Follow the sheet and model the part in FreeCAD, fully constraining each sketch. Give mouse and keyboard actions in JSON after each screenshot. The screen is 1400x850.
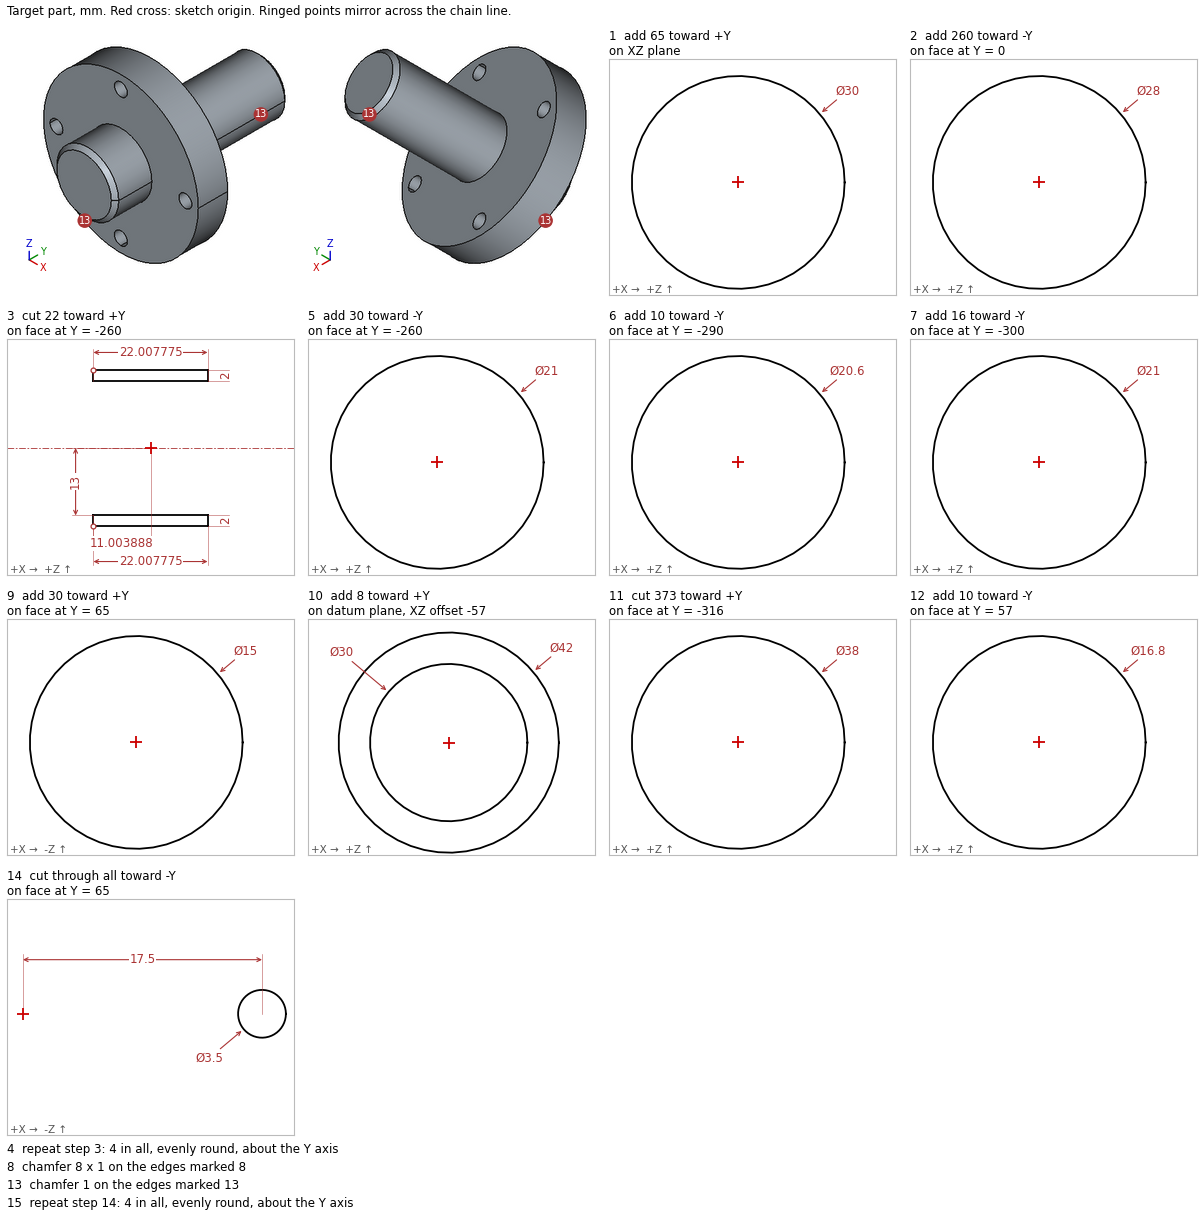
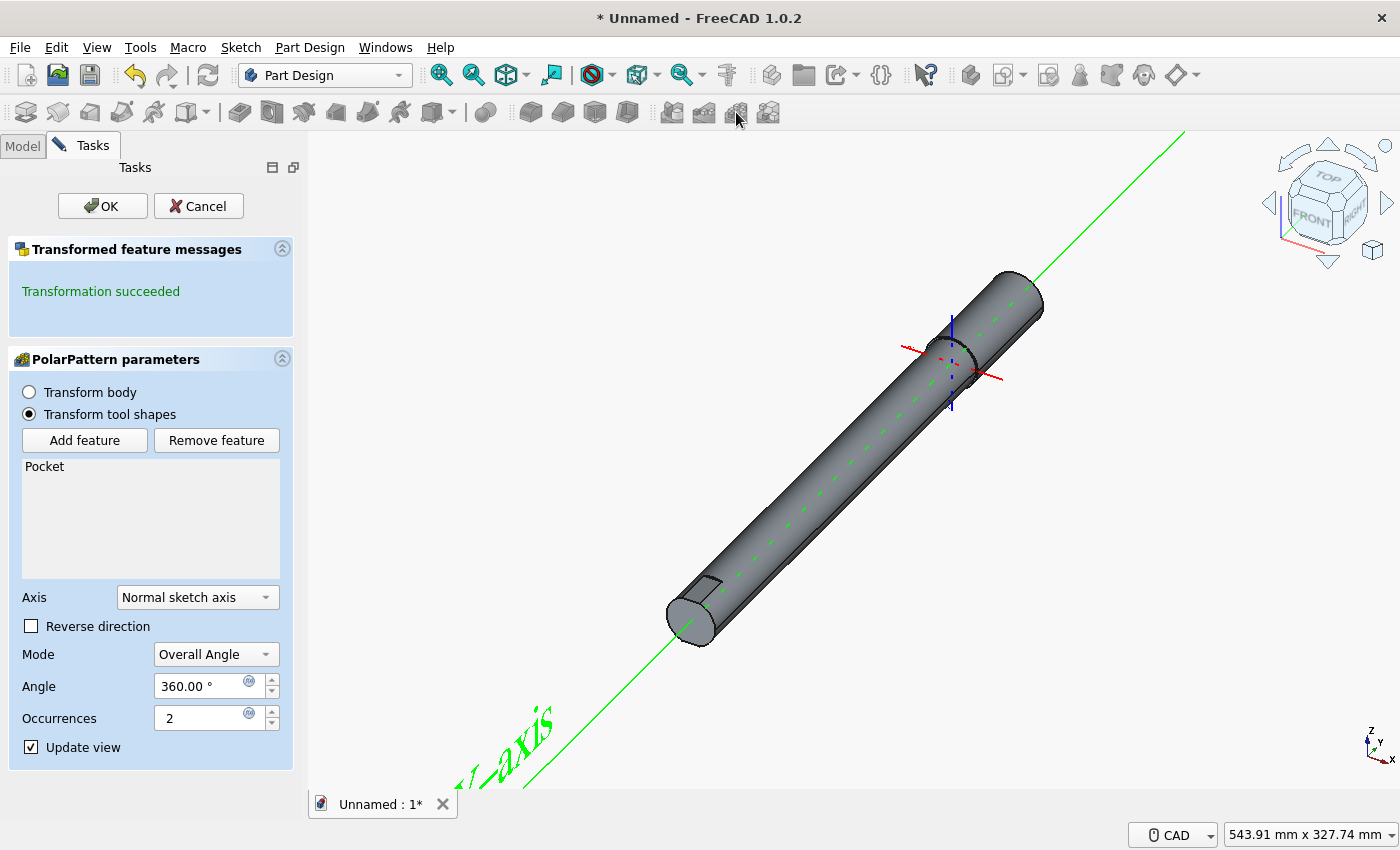
{"action": "left_click", "coordinate": [198, 598]}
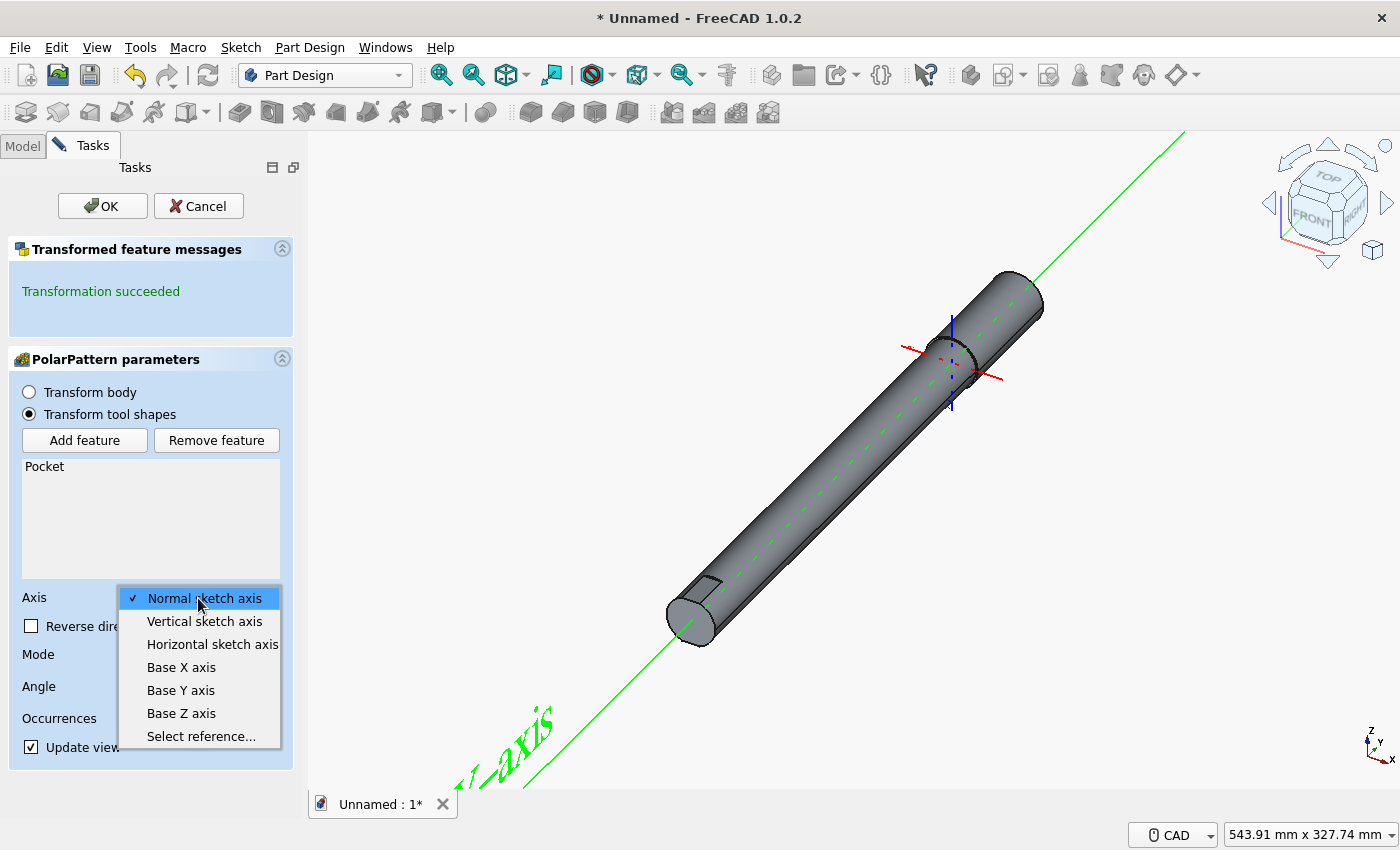
{"action": "left_click", "coordinate": [198, 690]}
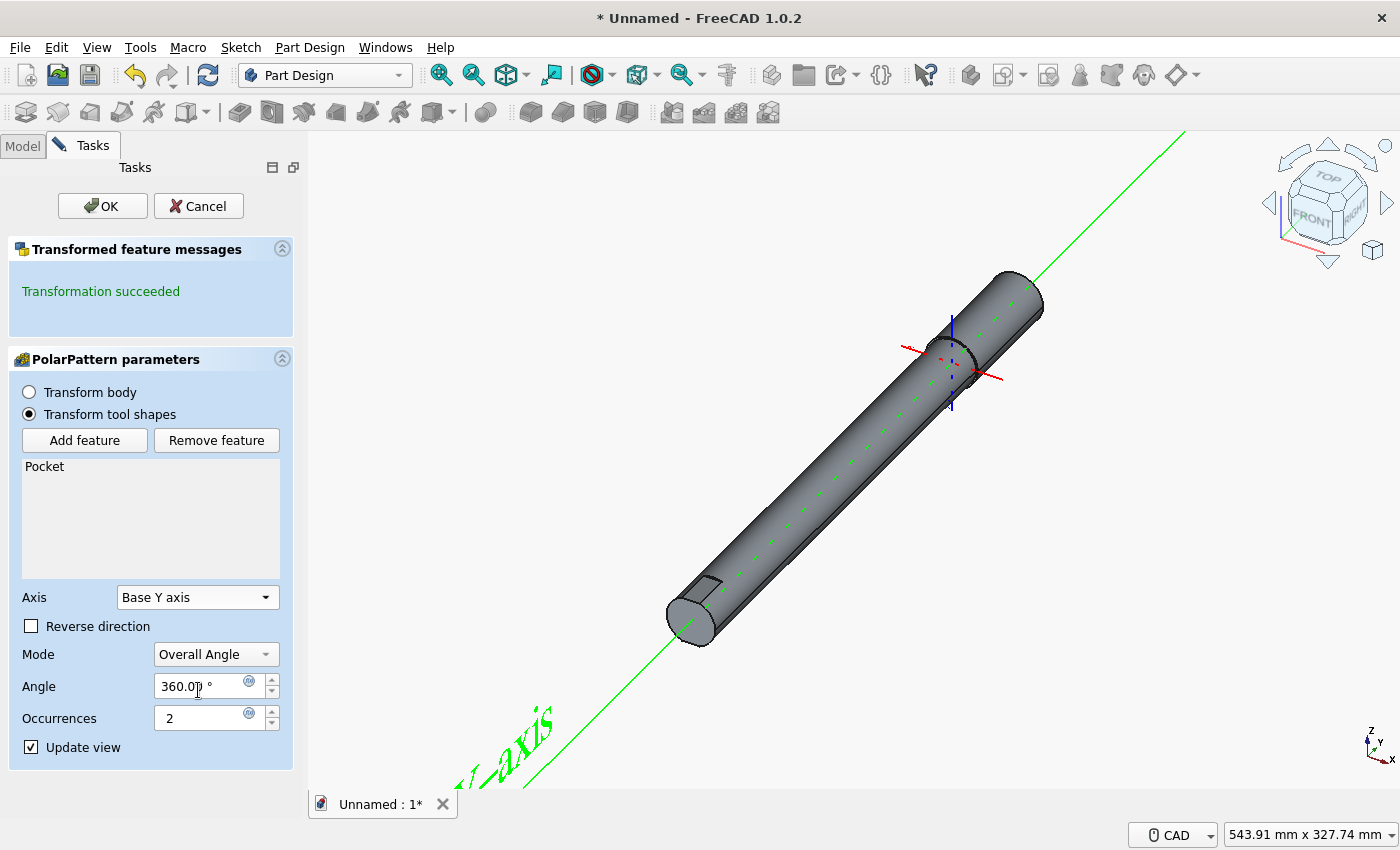
{"action": "triple_click", "coordinate": [209, 718]}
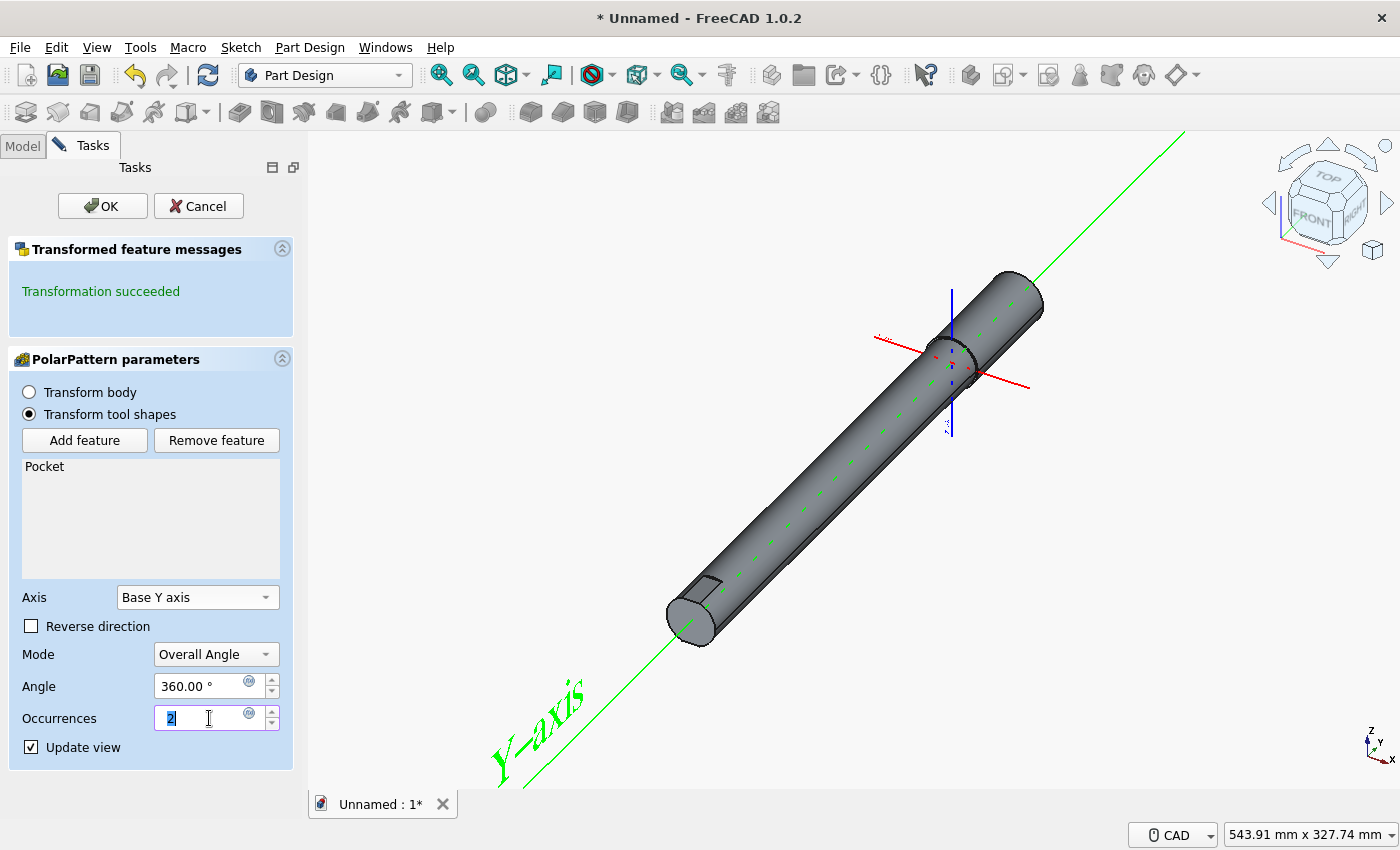
{"action": "type", "text": "4"}
{"action": "key", "text": "Tab"}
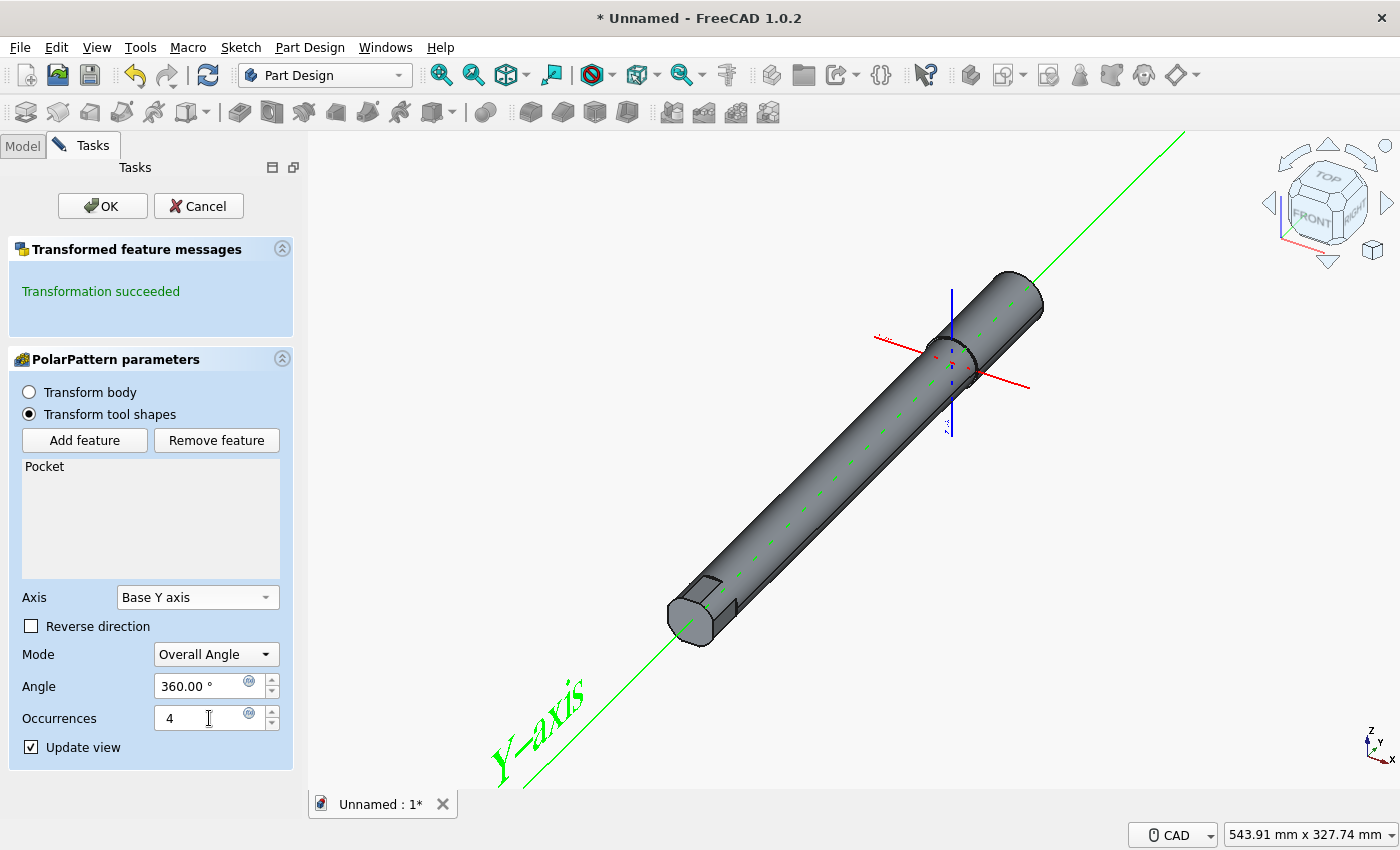
{"action": "left_click", "coordinate": [103, 206]}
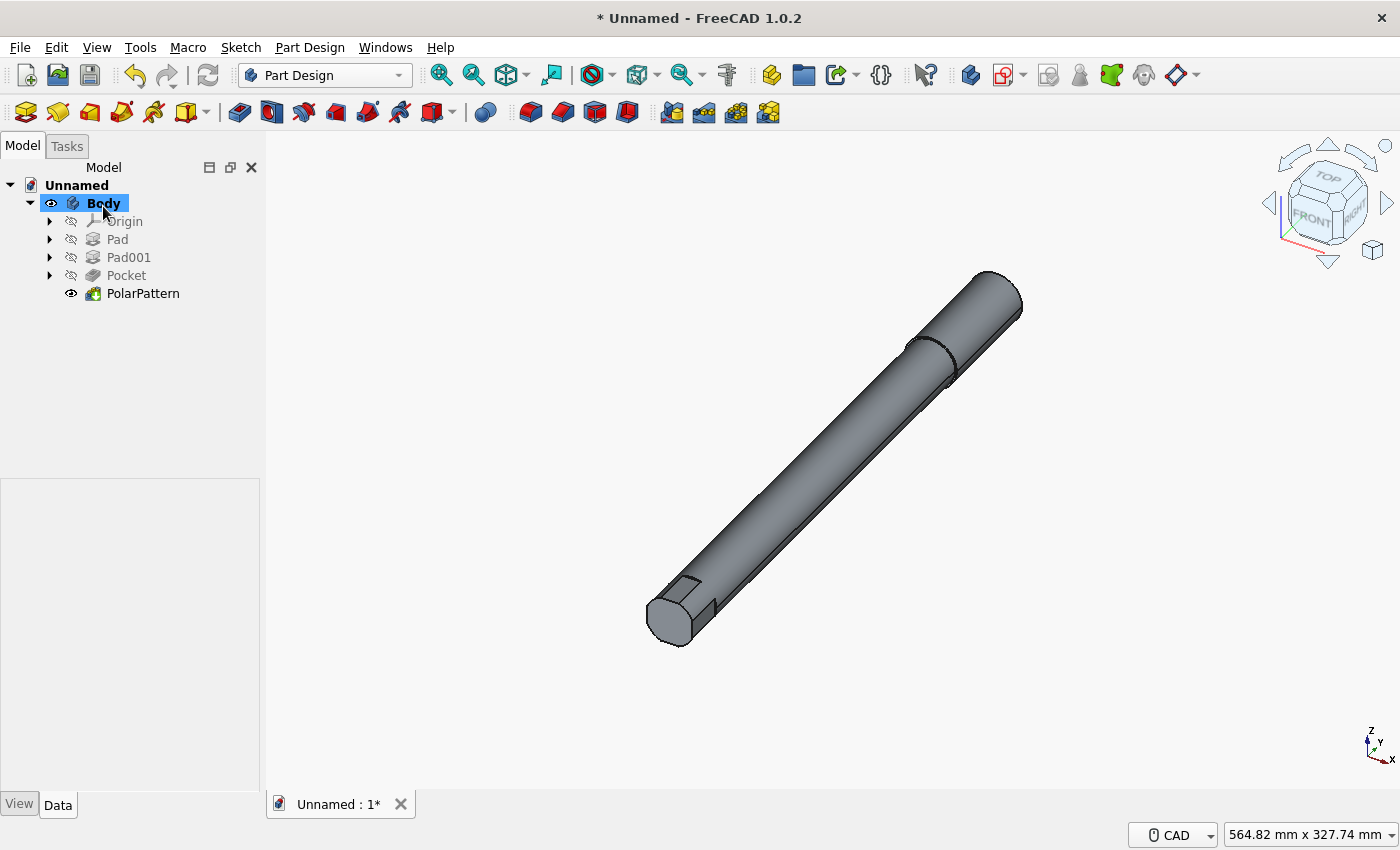
{"action": "left_click", "coordinate": [670, 621]}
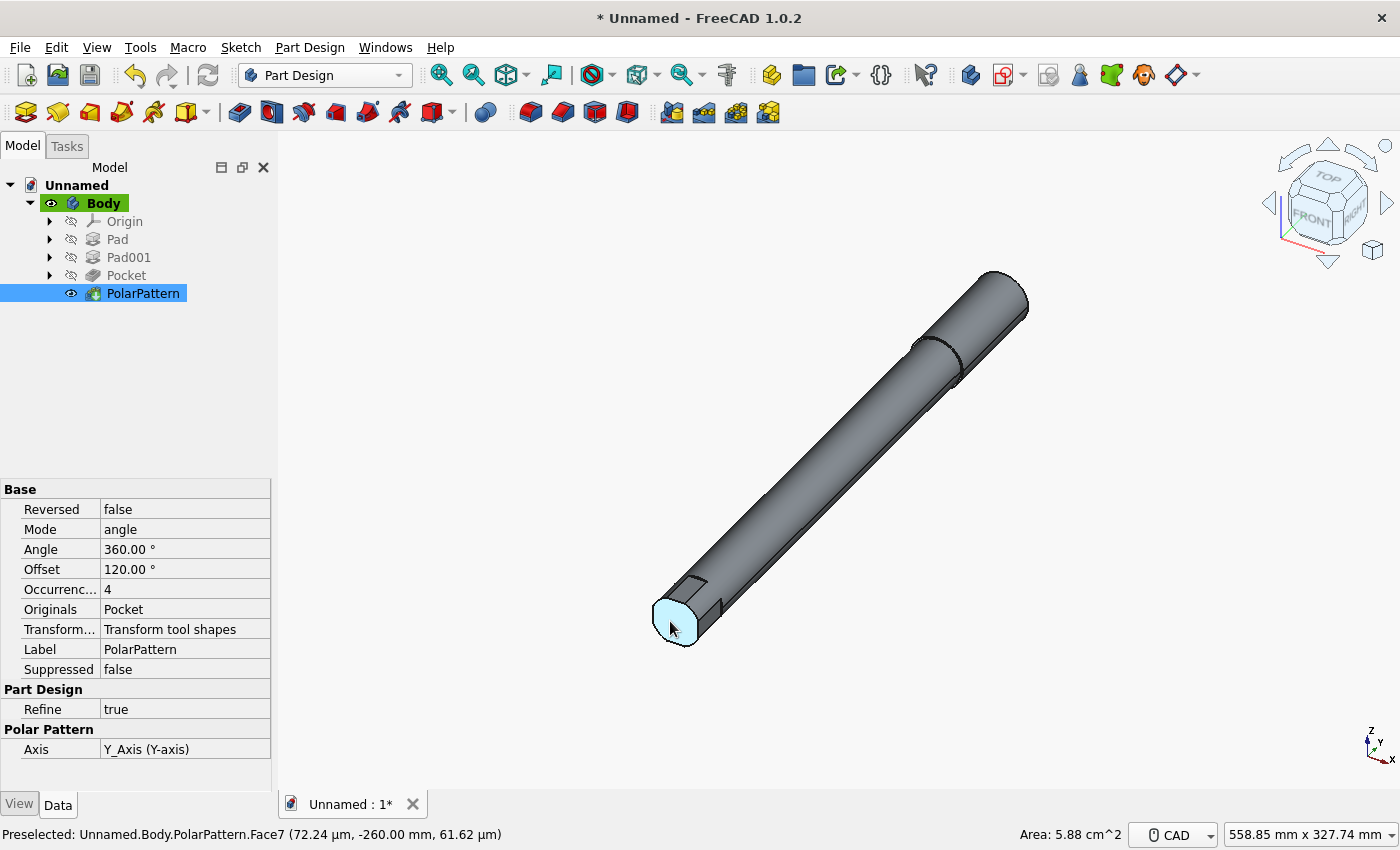
{"action": "left_click", "coordinate": [1004, 76]}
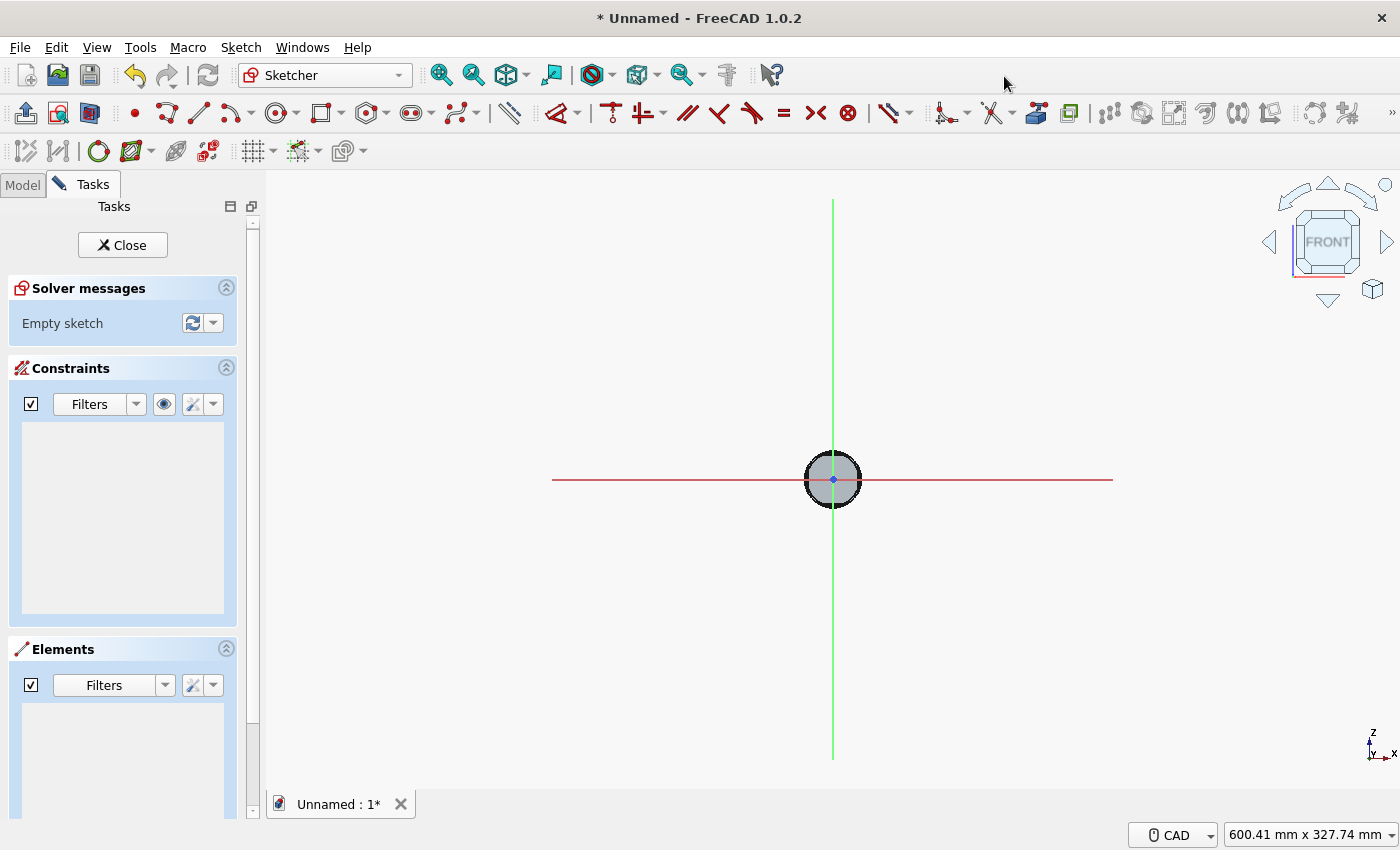
{"action": "scroll", "coordinate": [840, 480], "scroll_direction": "up", "scroll_amount": 12}